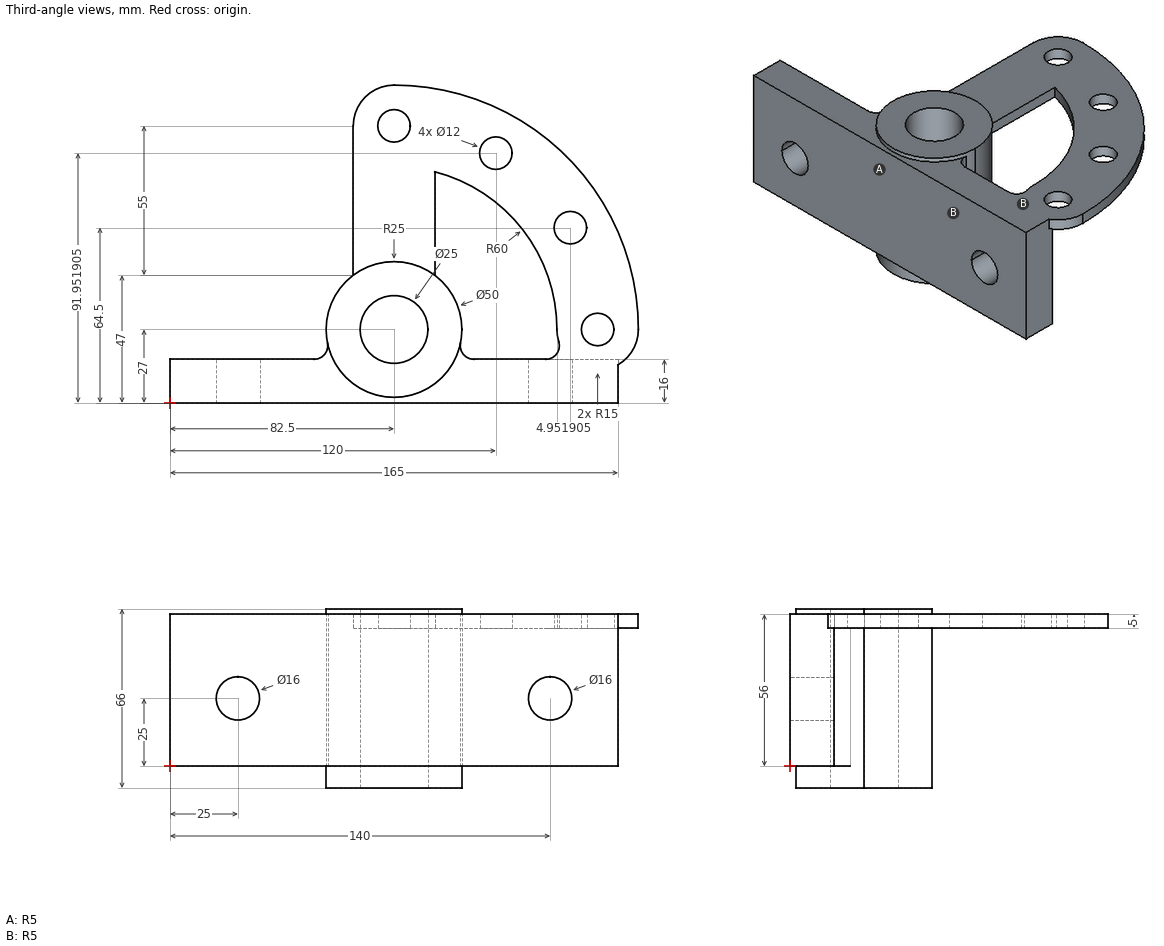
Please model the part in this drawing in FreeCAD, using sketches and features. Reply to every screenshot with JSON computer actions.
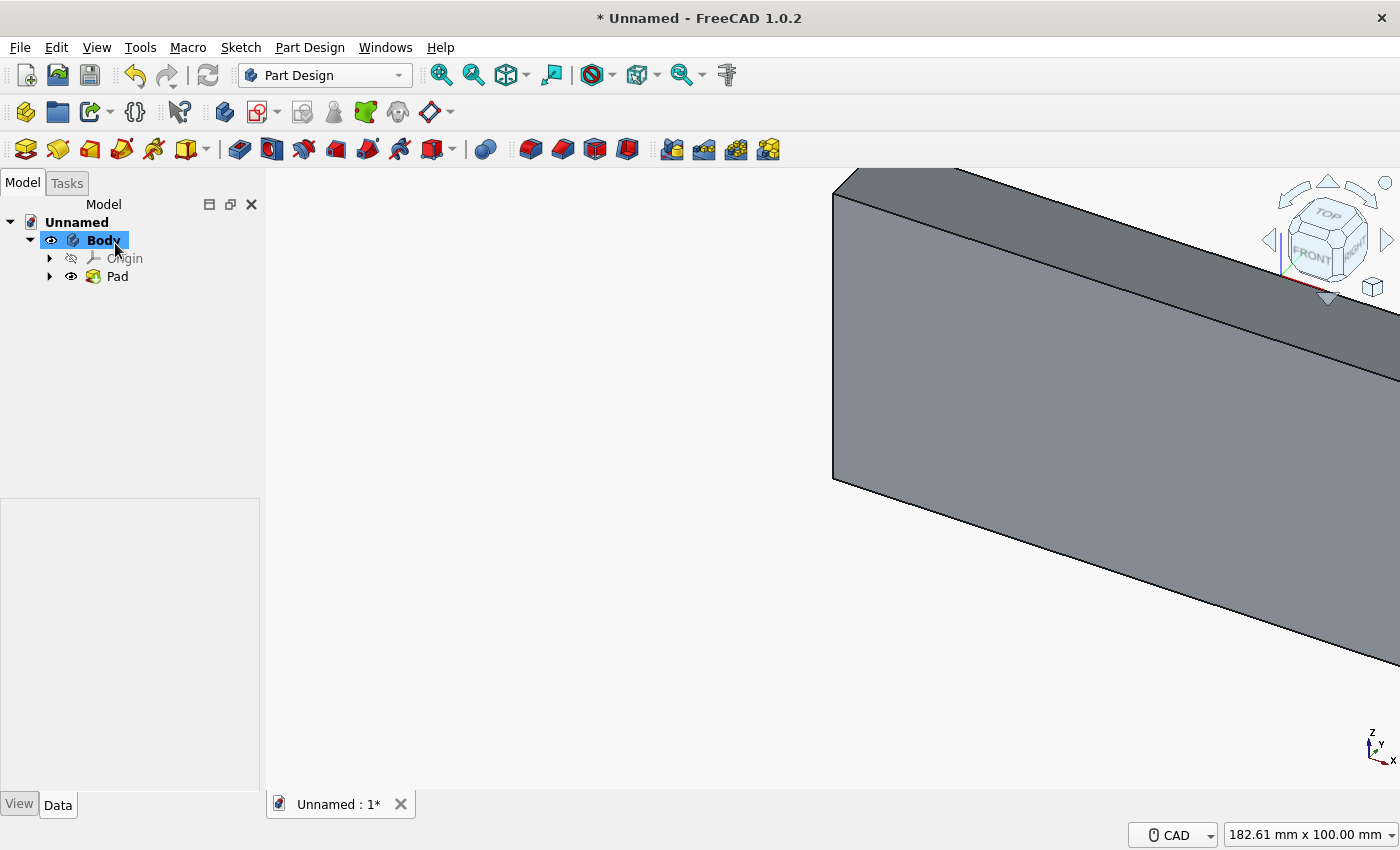
{"action": "left_click", "coordinate": [442, 76]}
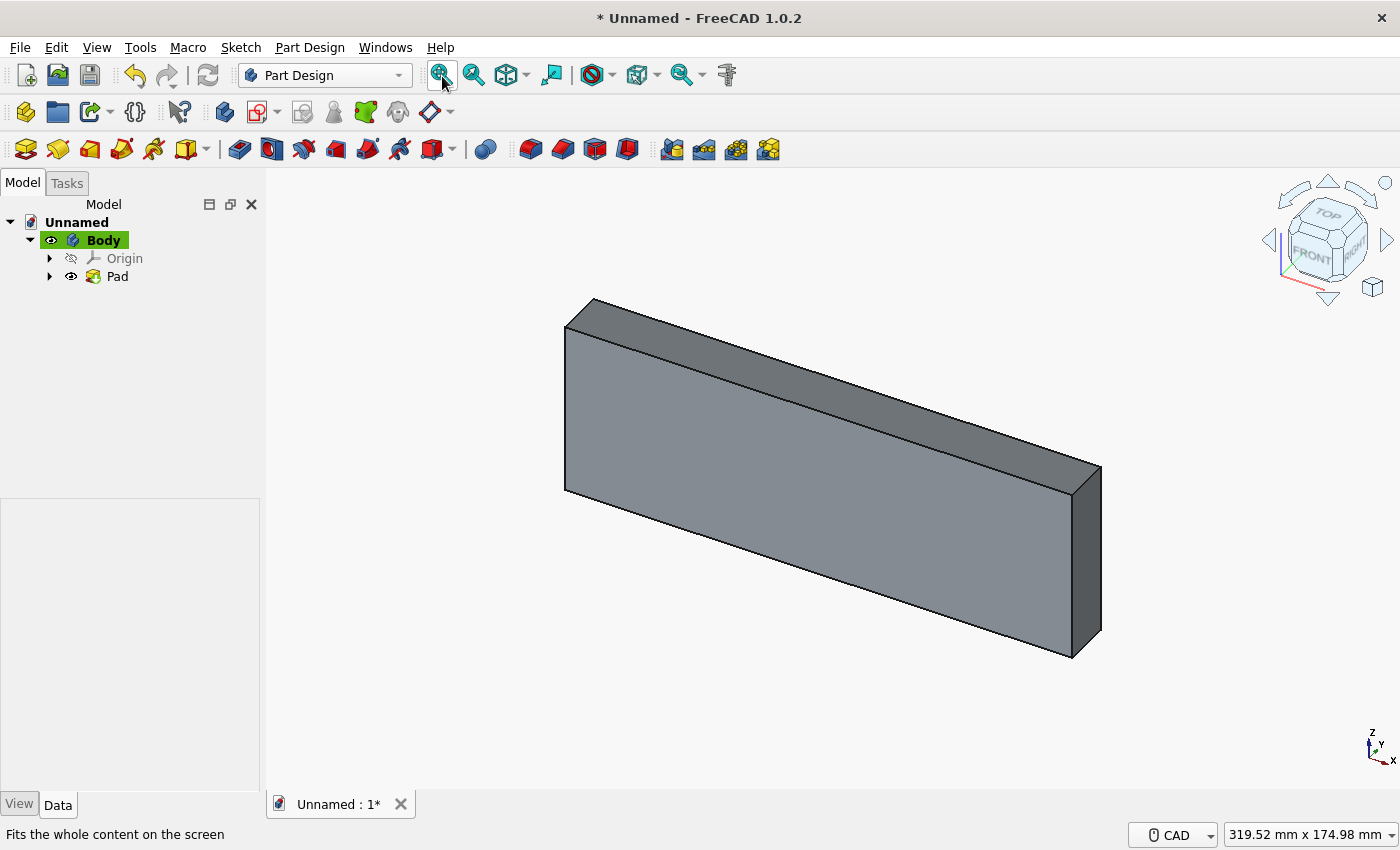
{"action": "left_click", "coordinate": [50, 258]}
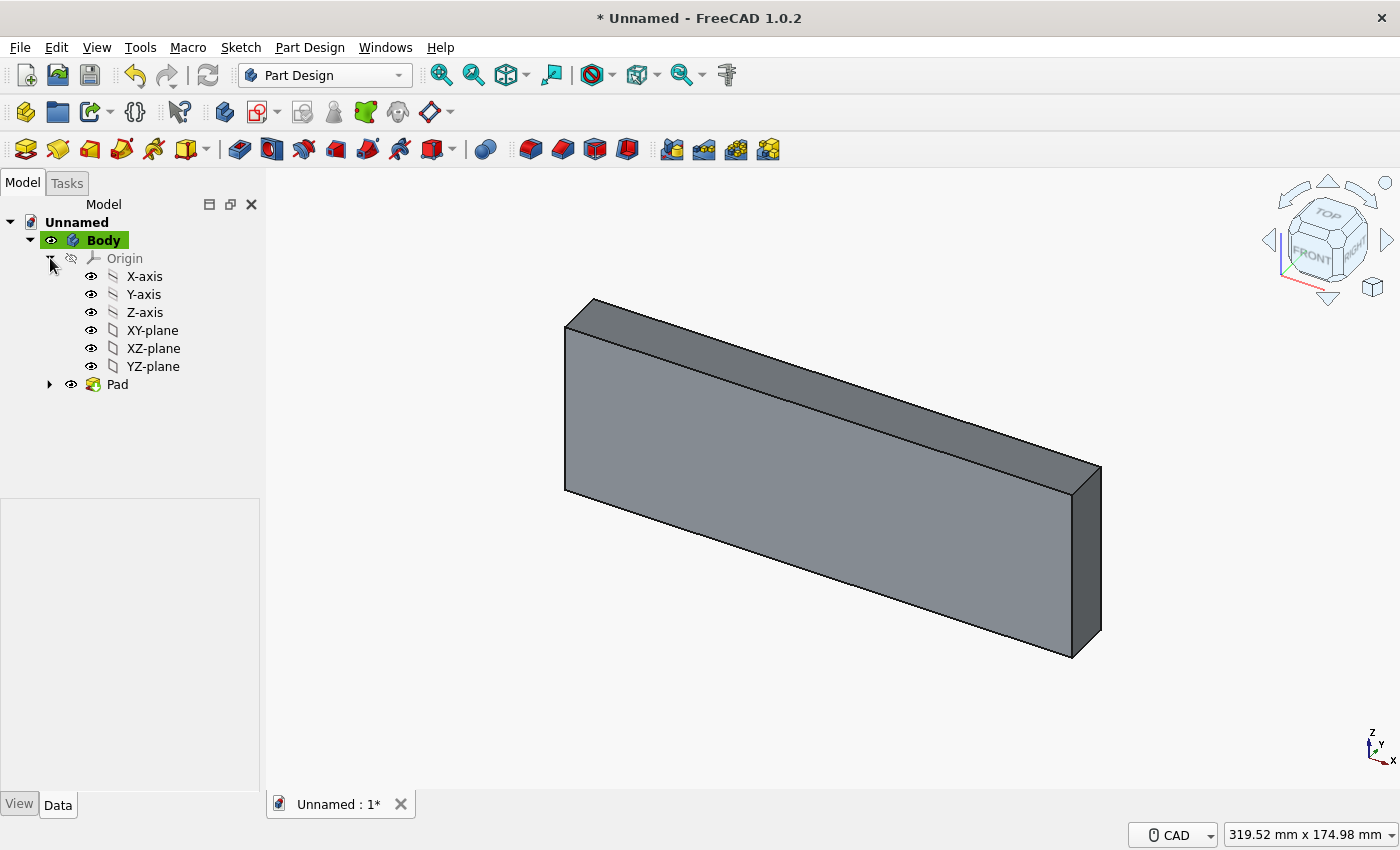
{"action": "left_click", "coordinate": [136, 330]}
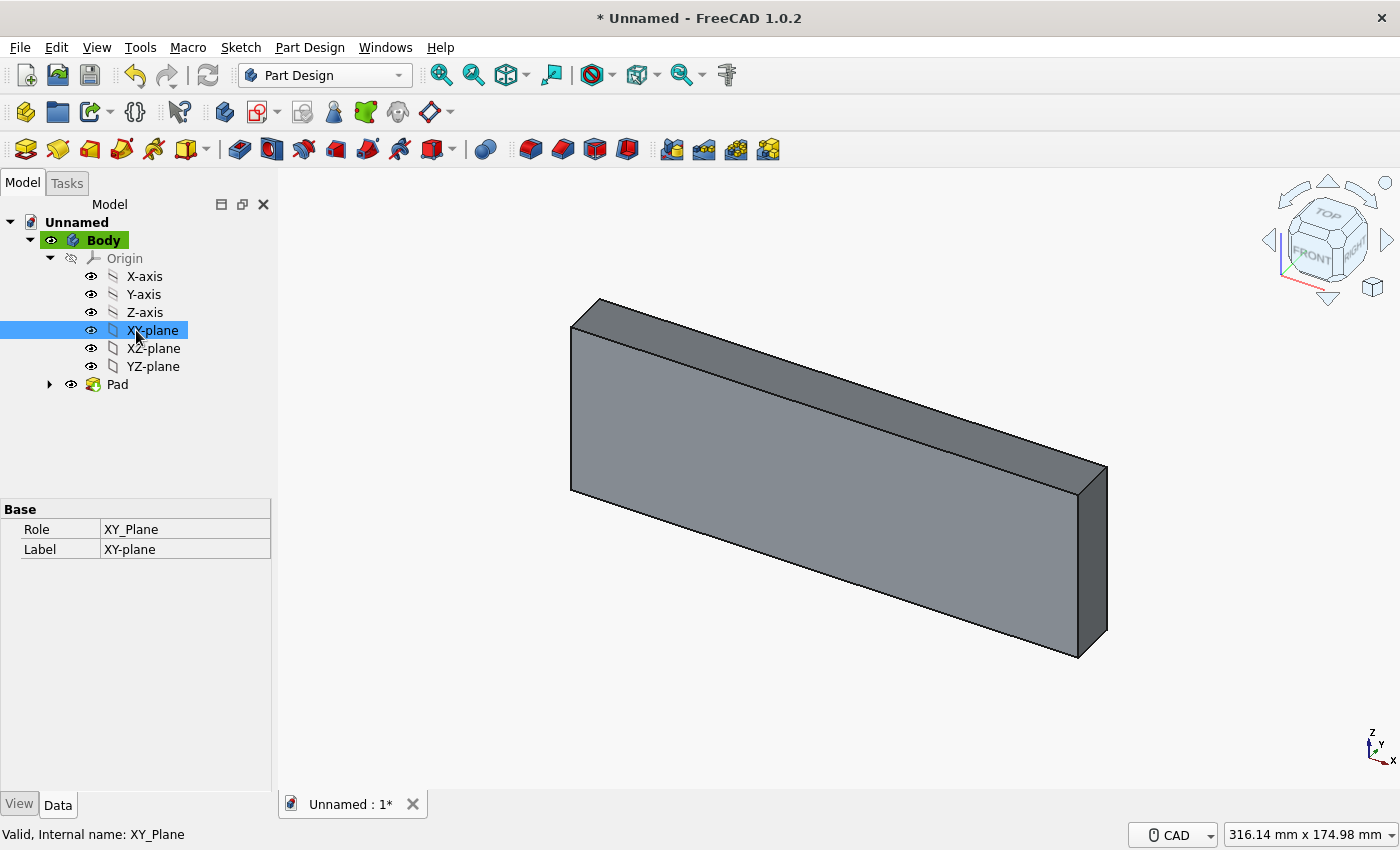
{"action": "left_click", "coordinate": [430, 112]}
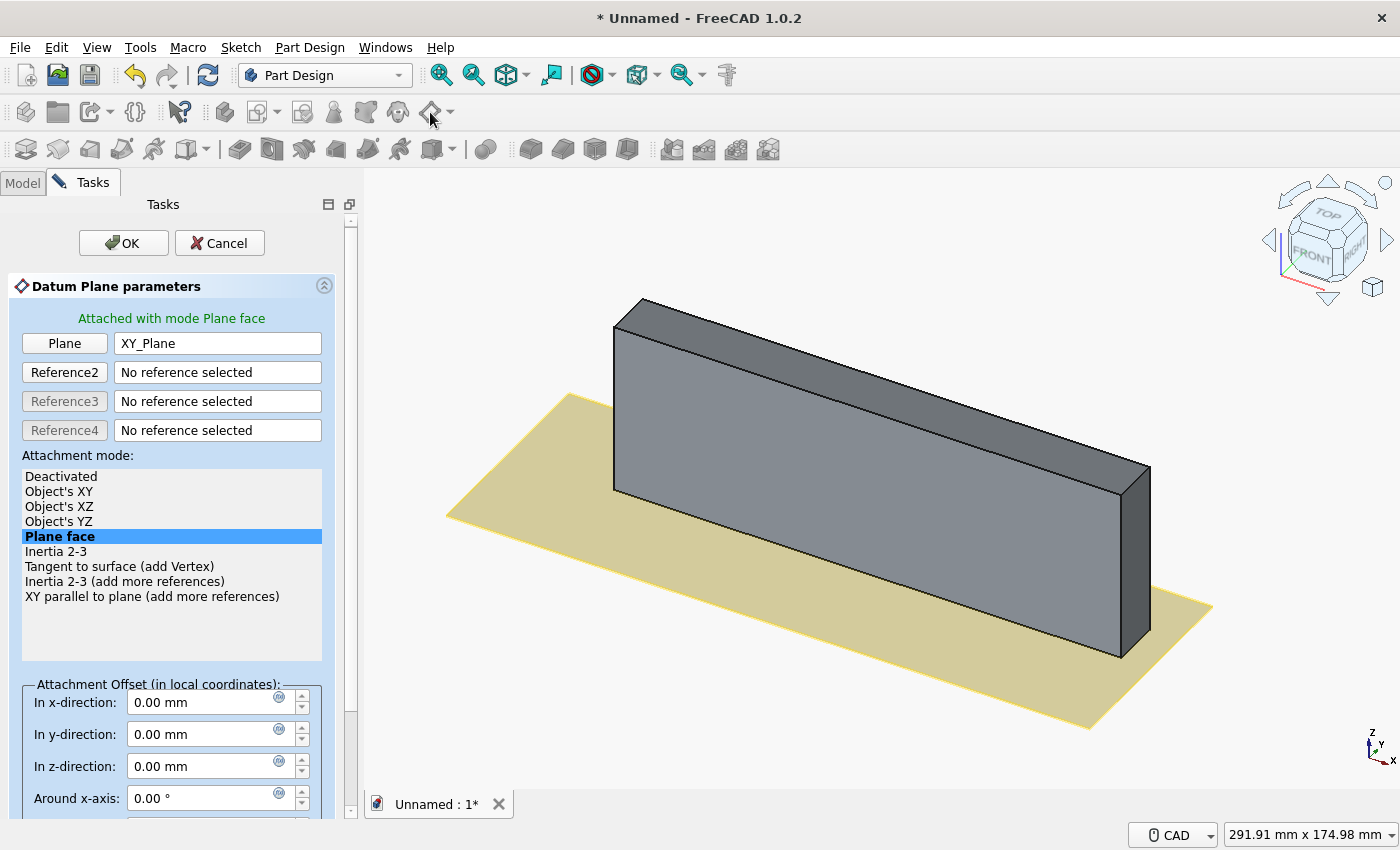
{"action": "triple_click", "coordinate": [210, 766]}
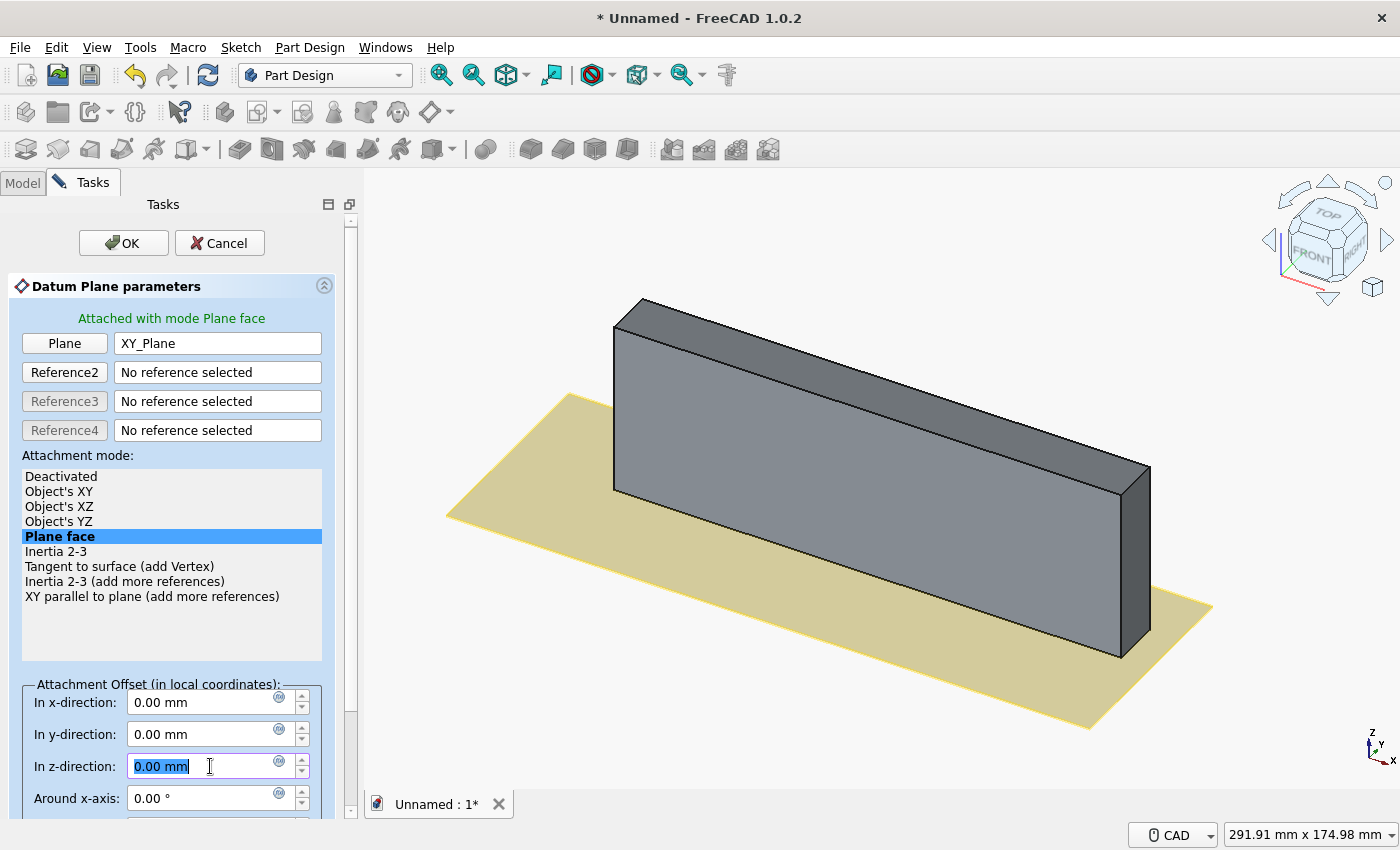
{"action": "type", "text": "25"}
{"action": "key", "text": "Tab"}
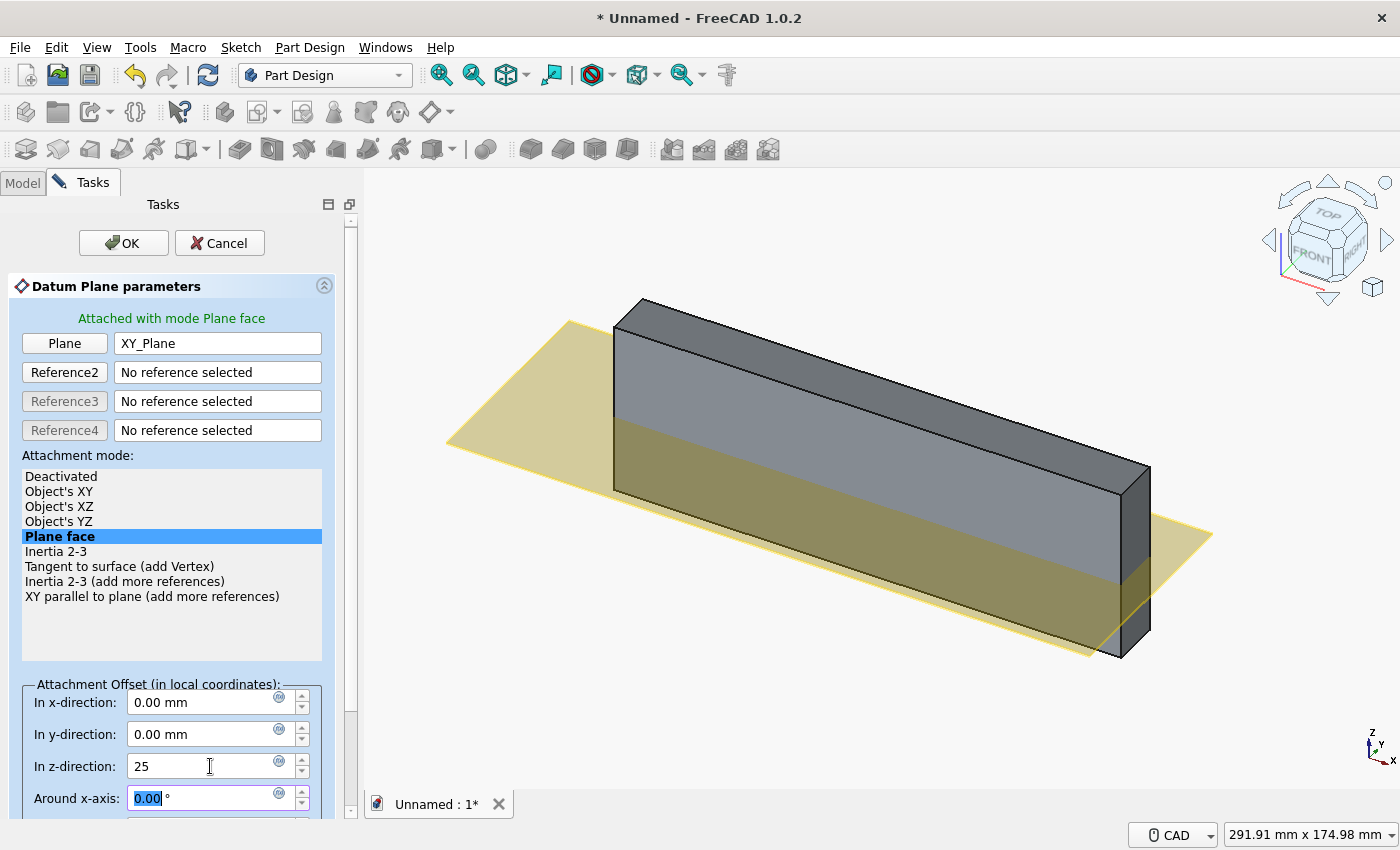
{"action": "left_click", "coordinate": [124, 243]}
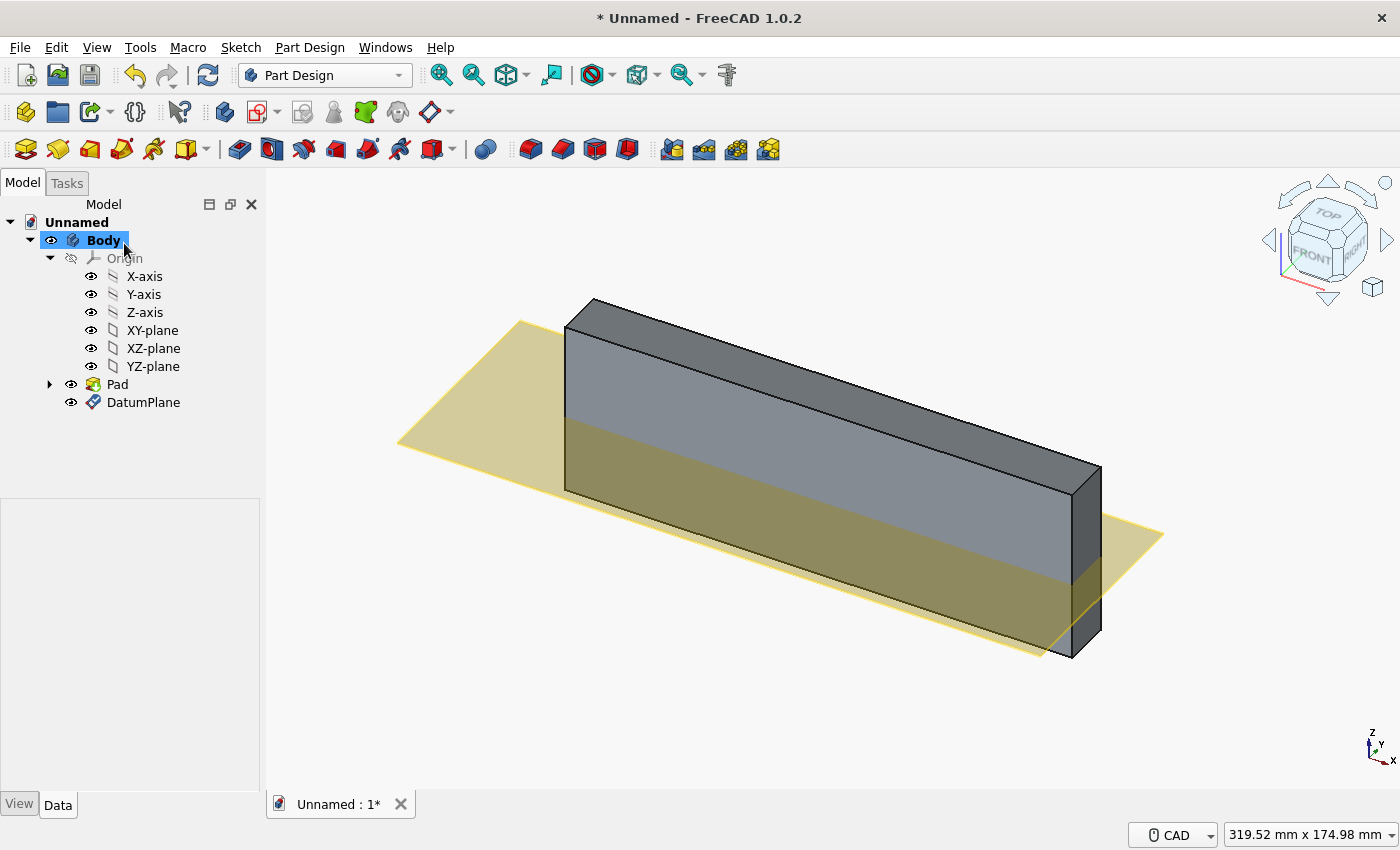
{"action": "left_click", "coordinate": [116, 402]}